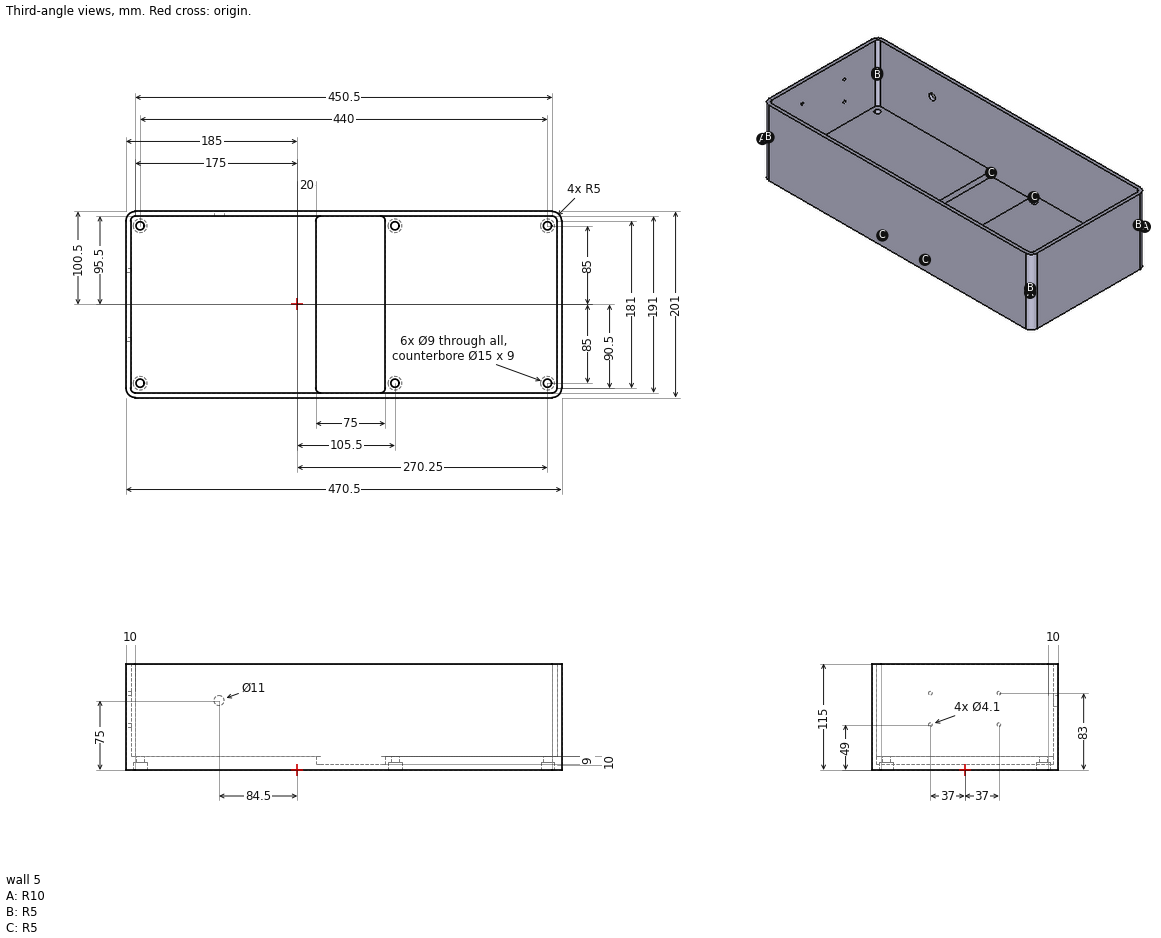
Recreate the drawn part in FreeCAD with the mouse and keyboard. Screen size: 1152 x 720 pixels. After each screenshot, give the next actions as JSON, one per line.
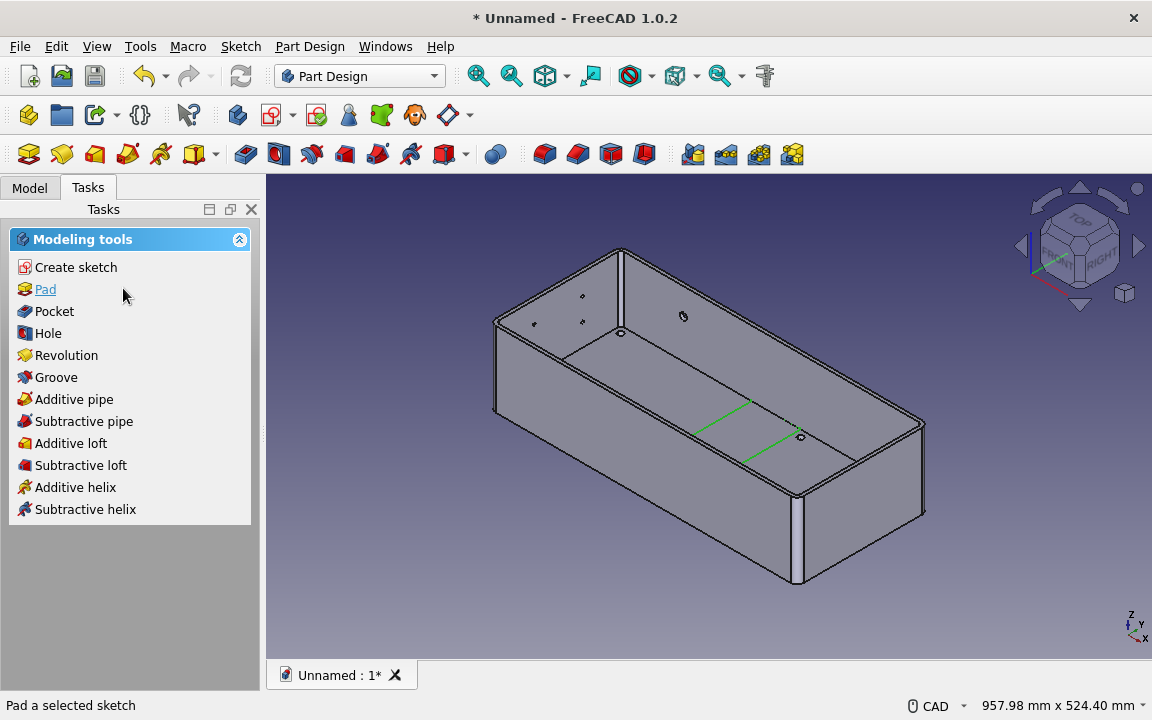
{"action": "left_click", "coordinate": [246, 154]}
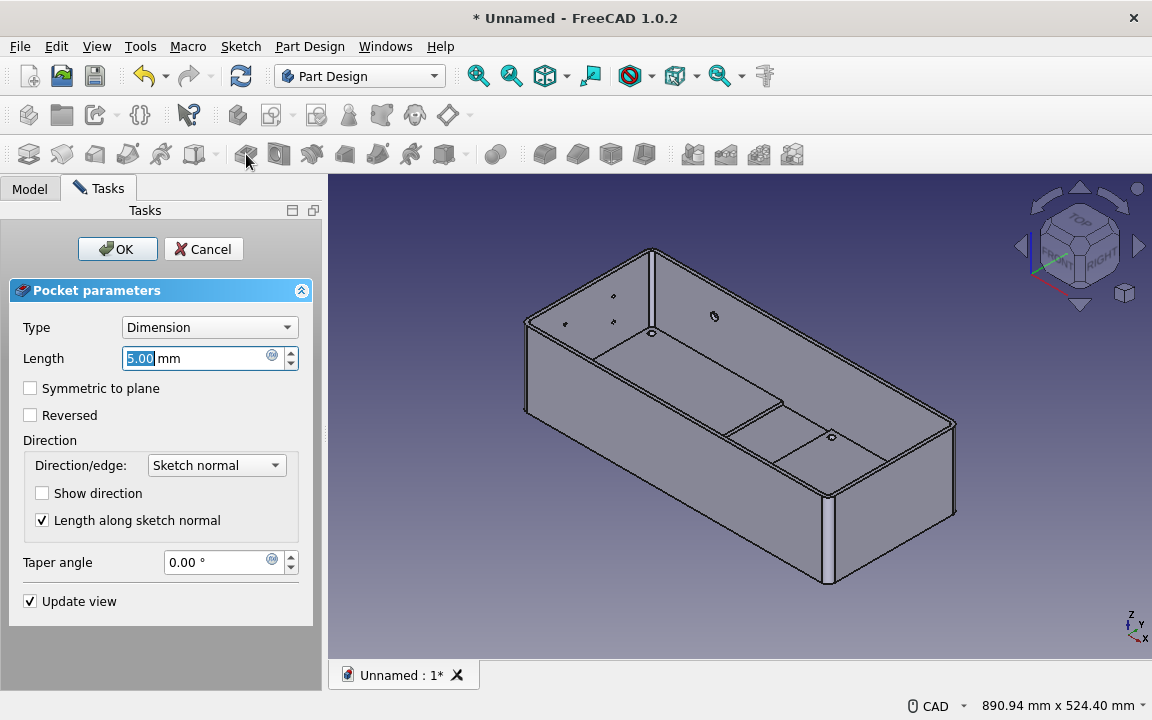
{"action": "type", "text": "9"}
{"action": "key", "text": "Tab"}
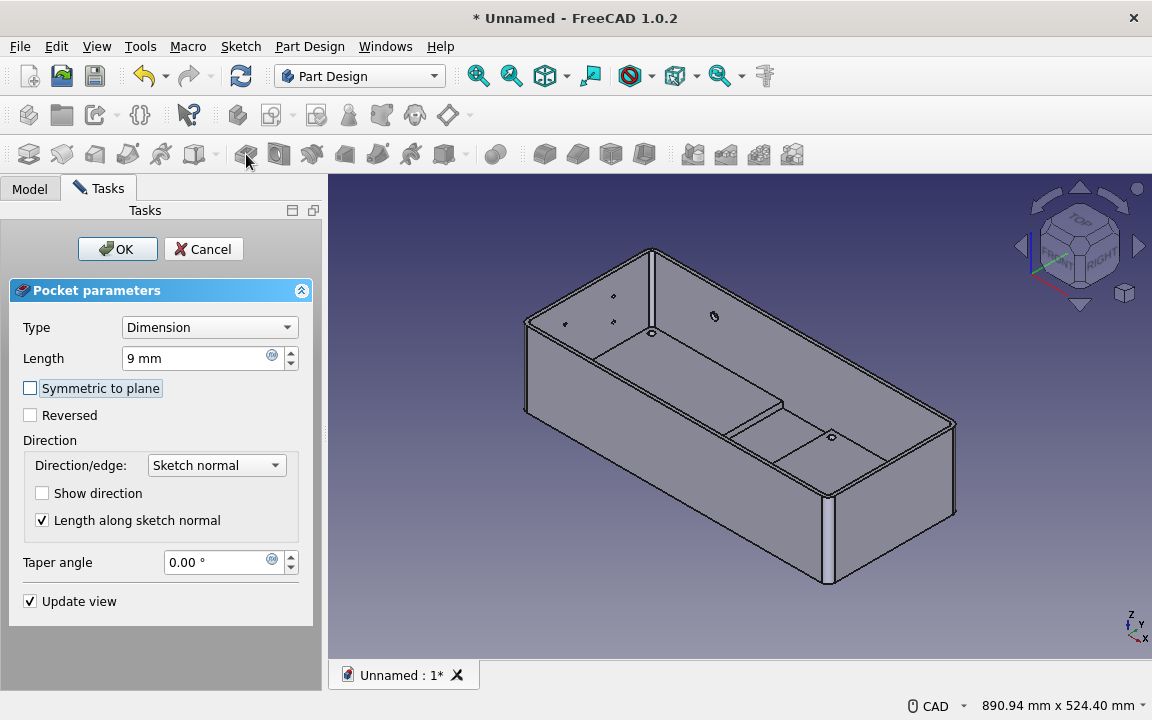
{"action": "left_click", "coordinate": [118, 249]}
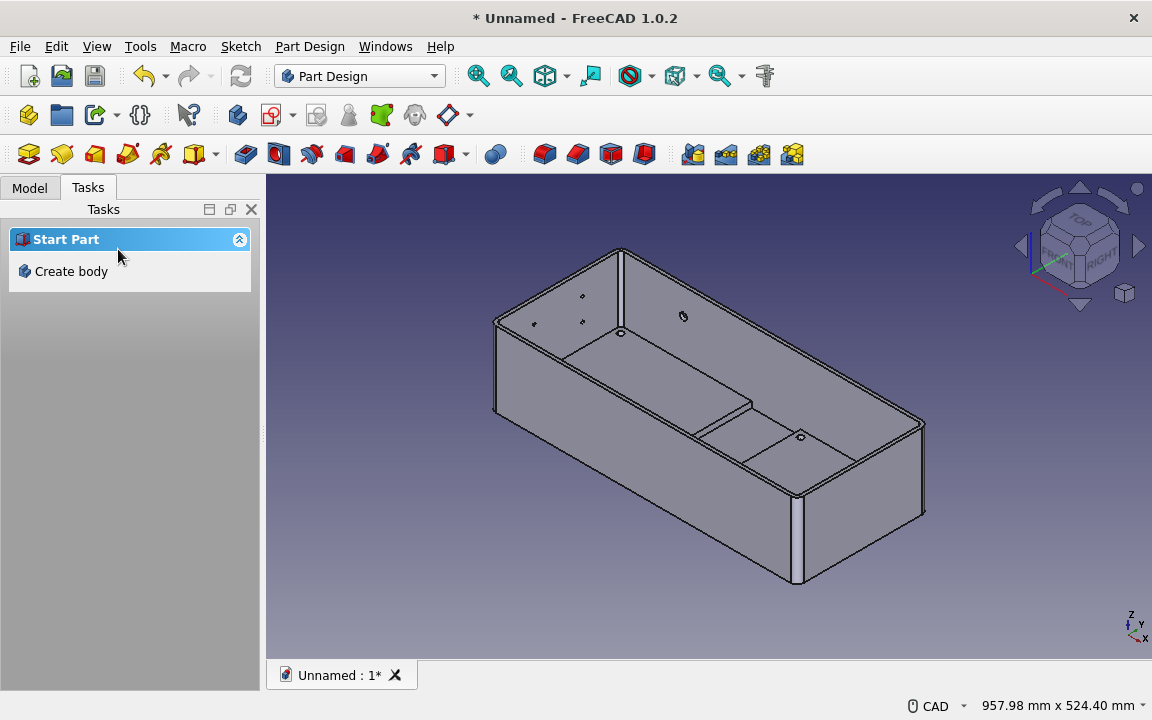
{"action": "scroll", "coordinate": [627, 476], "scroll_direction": "up", "scroll_amount": 8}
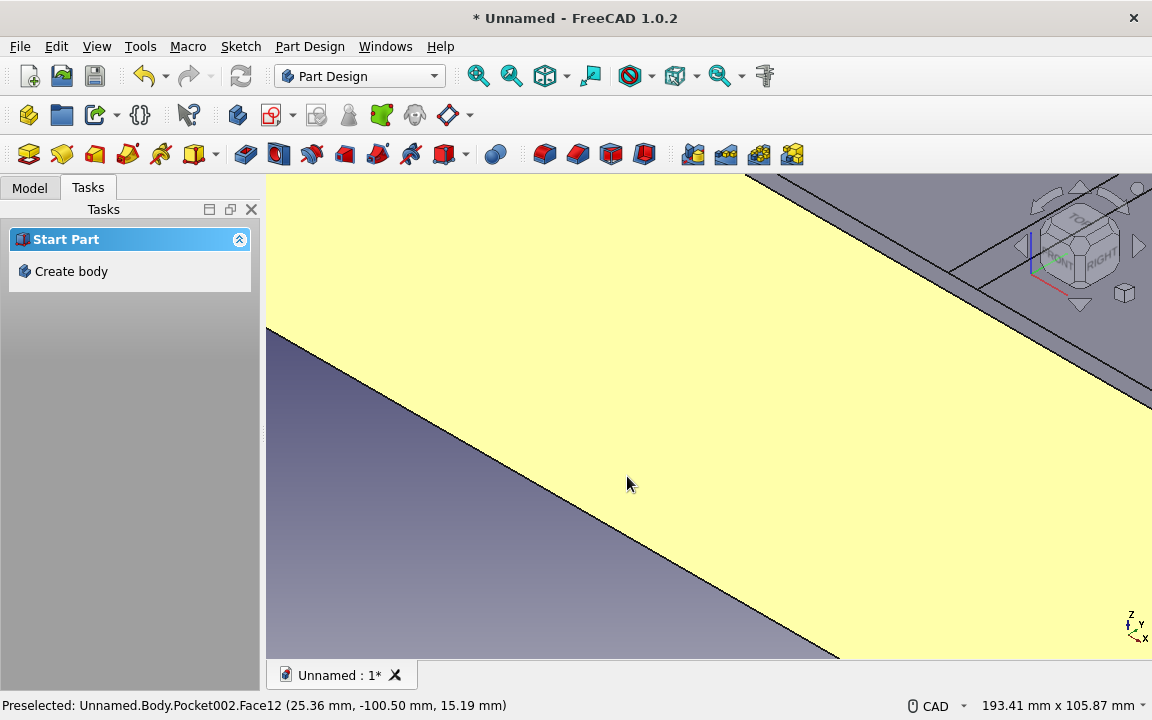
{"action": "key", "text": "v f"}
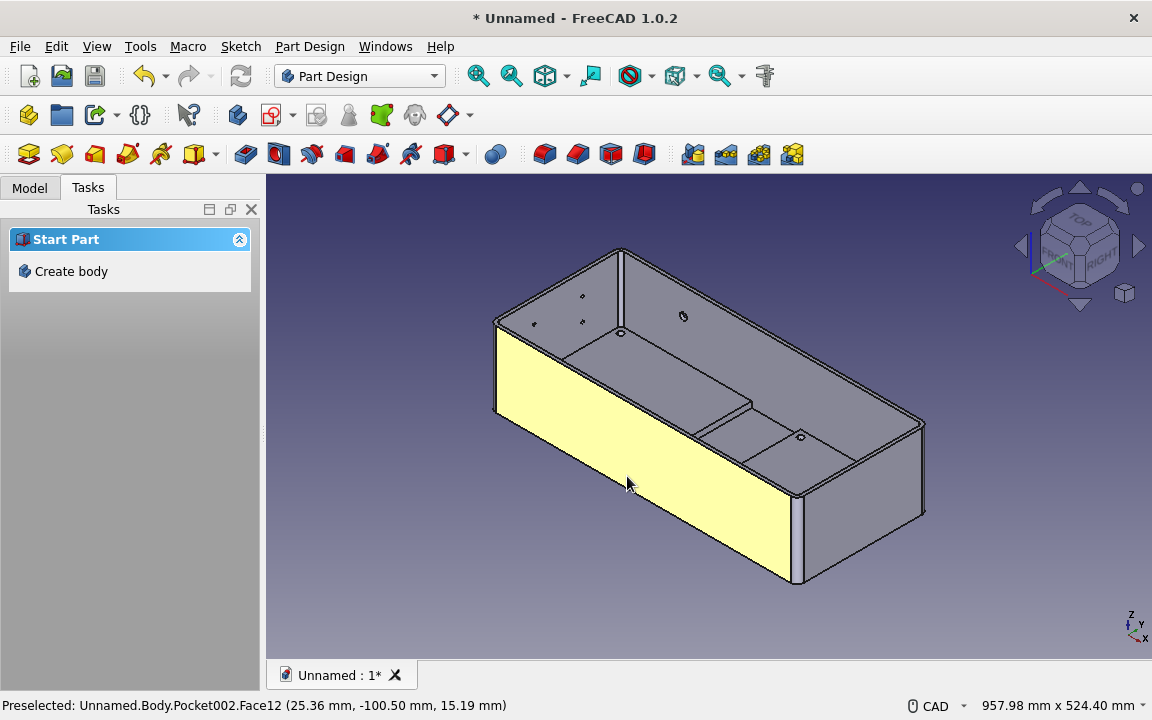
{"action": "key", "text": "2"}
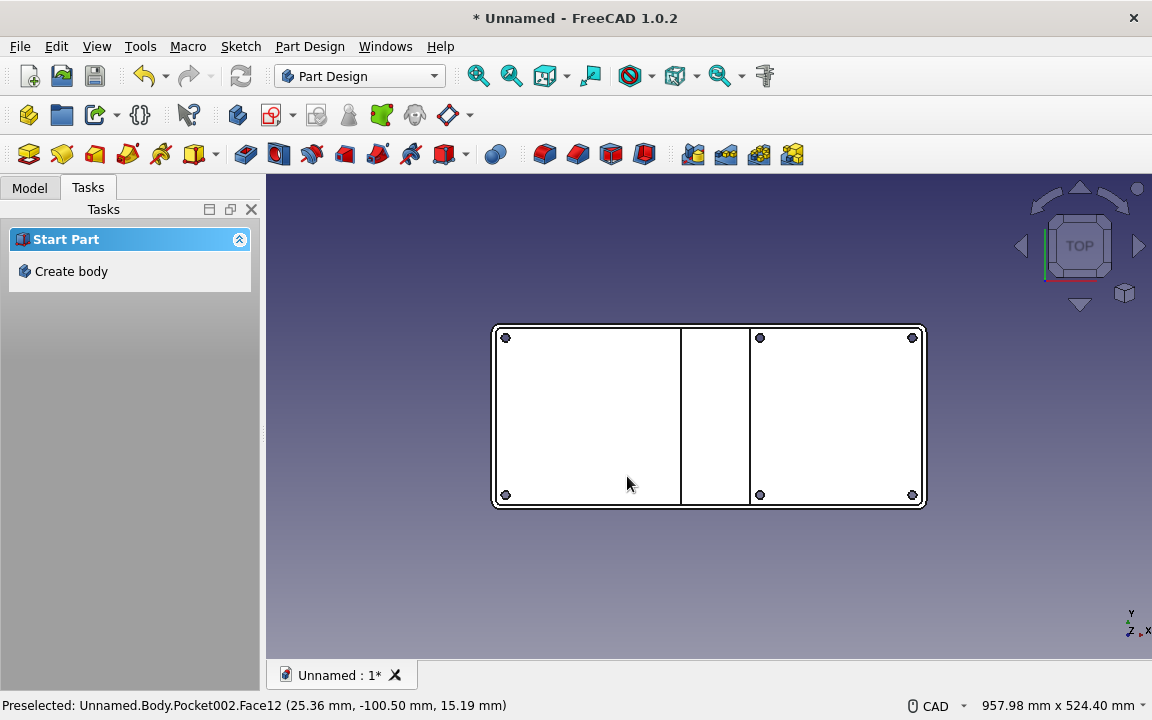
{"action": "scroll", "coordinate": [681, 504], "scroll_direction": "up", "scroll_amount": 8}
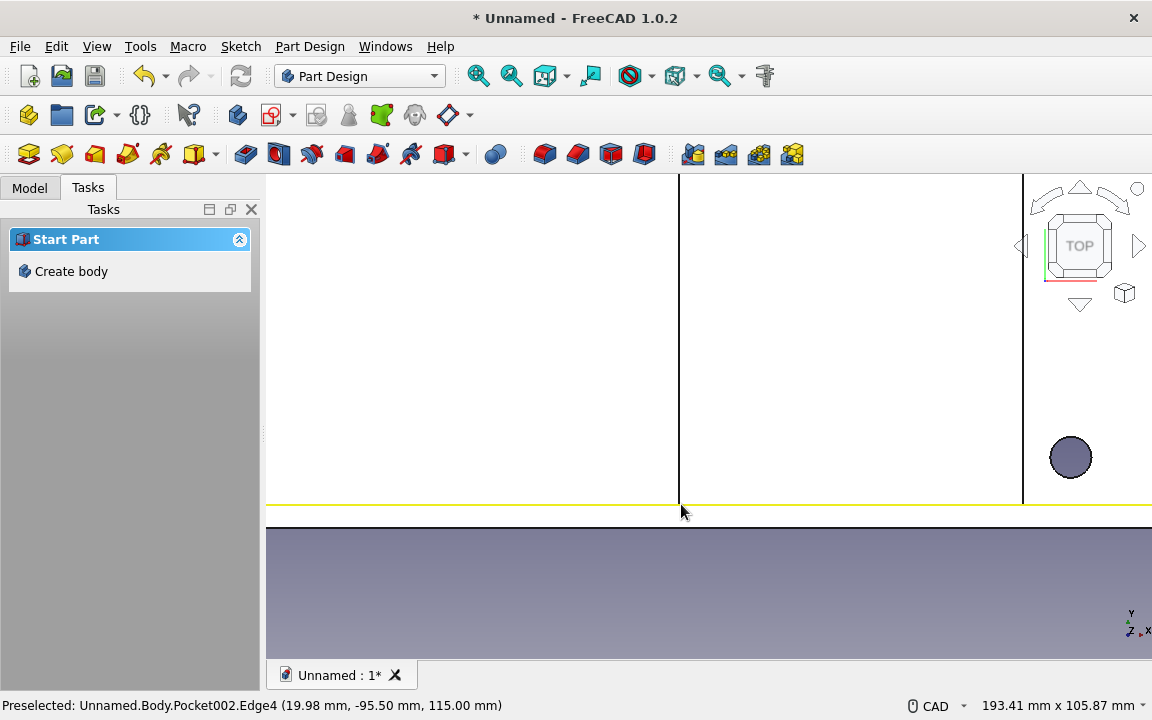
{"action": "key", "text": "v f"}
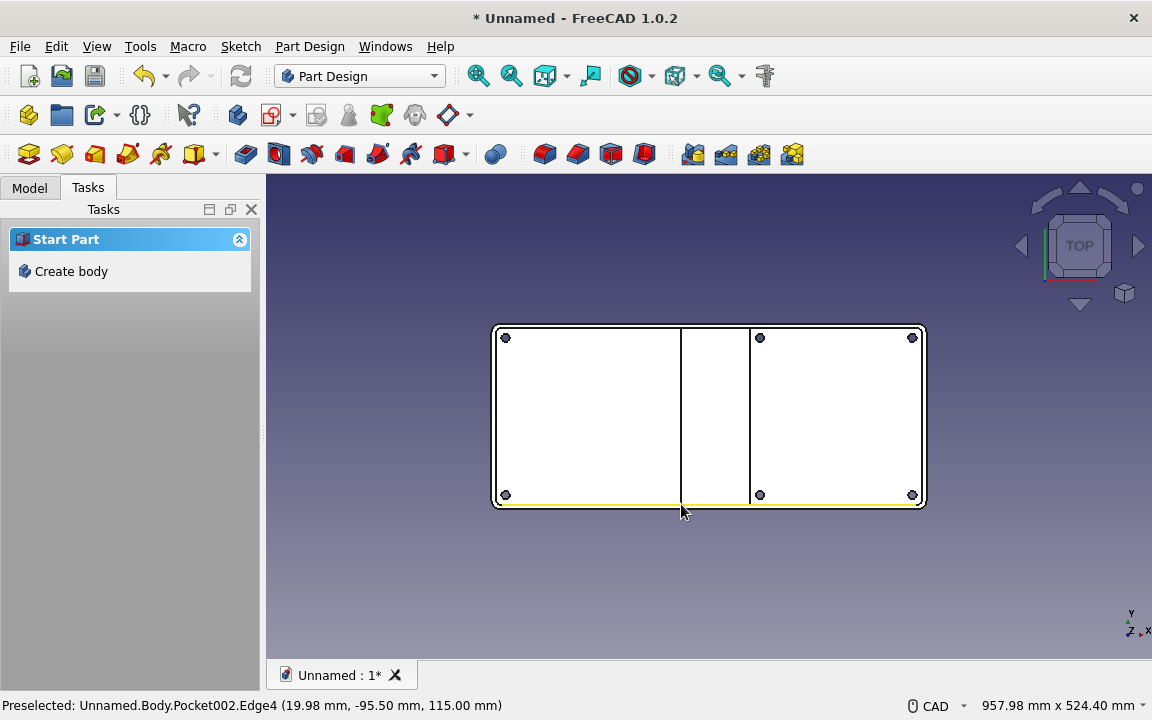
{"action": "key", "text": "0"}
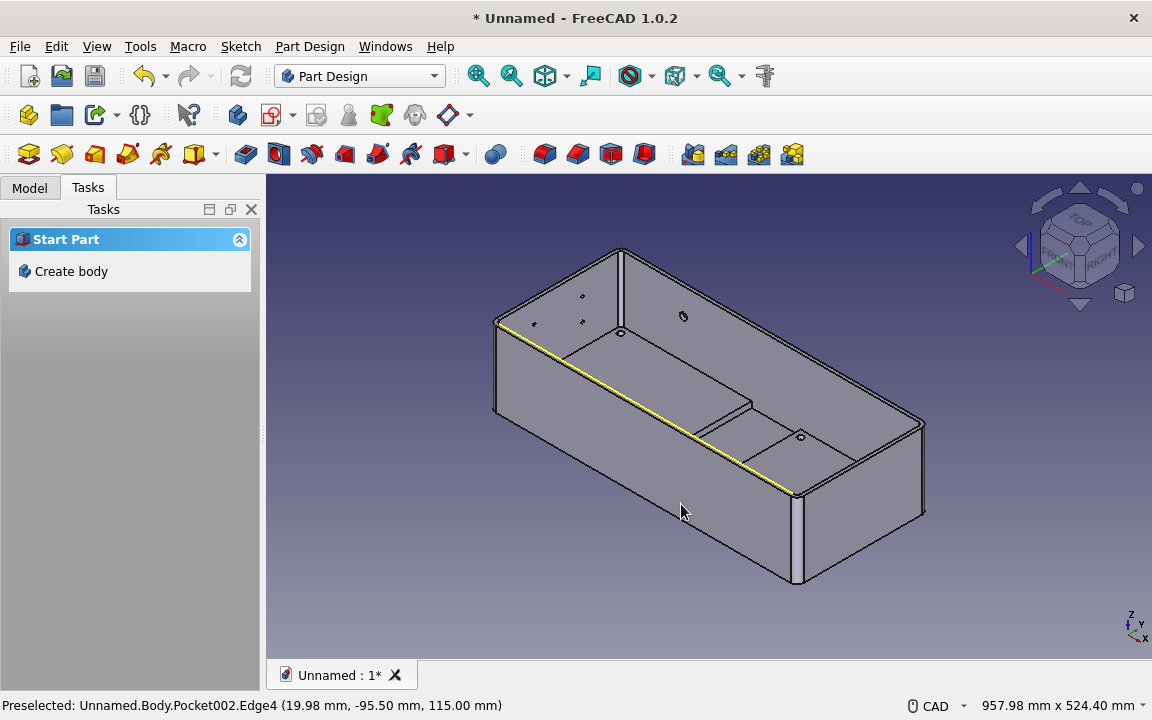
{"action": "scroll", "coordinate": [627, 476], "scroll_direction": "up", "scroll_amount": 8}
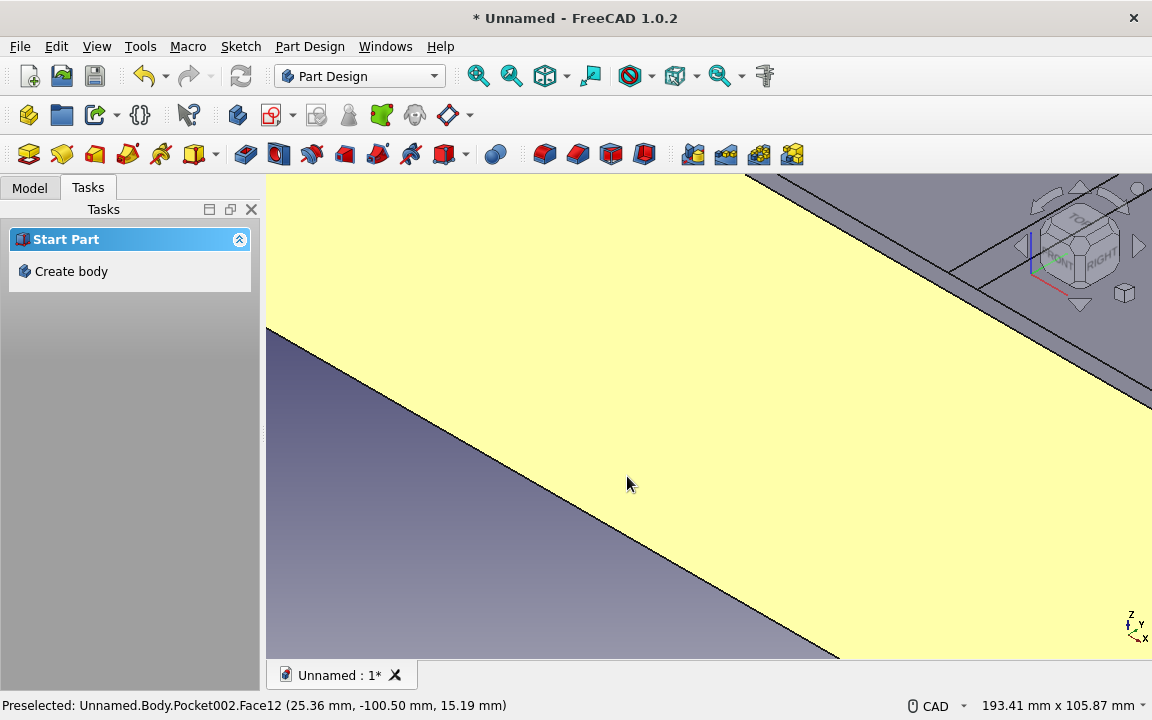
{"action": "key", "text": "v f"}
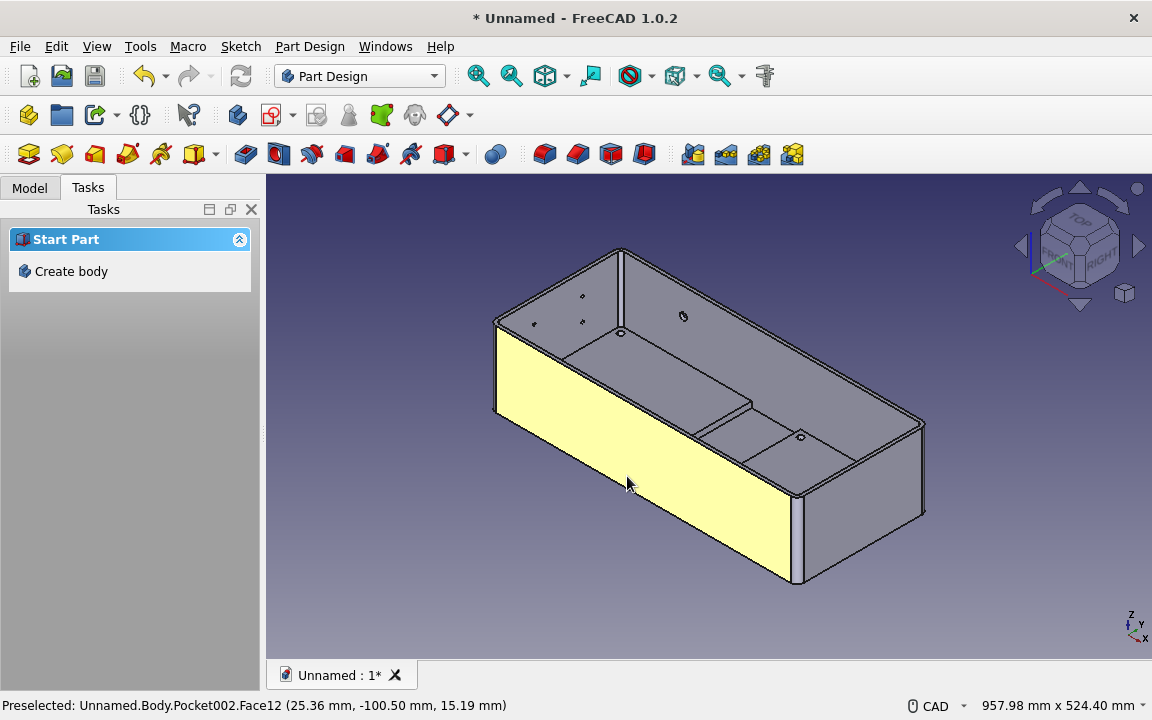
{"action": "key", "text": "1"}